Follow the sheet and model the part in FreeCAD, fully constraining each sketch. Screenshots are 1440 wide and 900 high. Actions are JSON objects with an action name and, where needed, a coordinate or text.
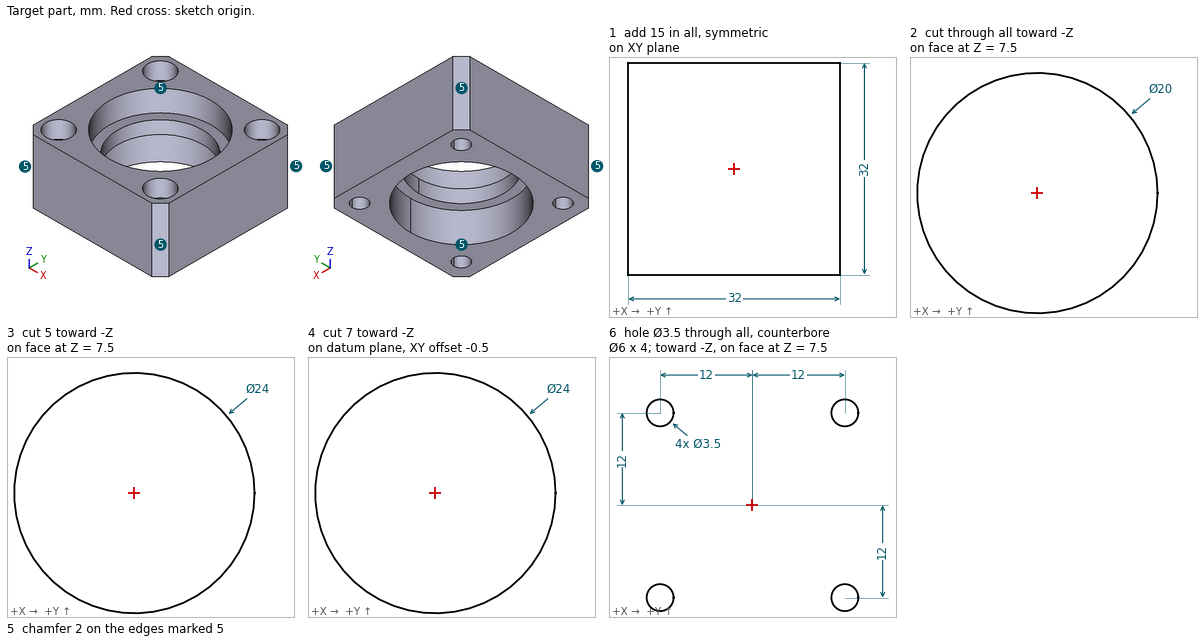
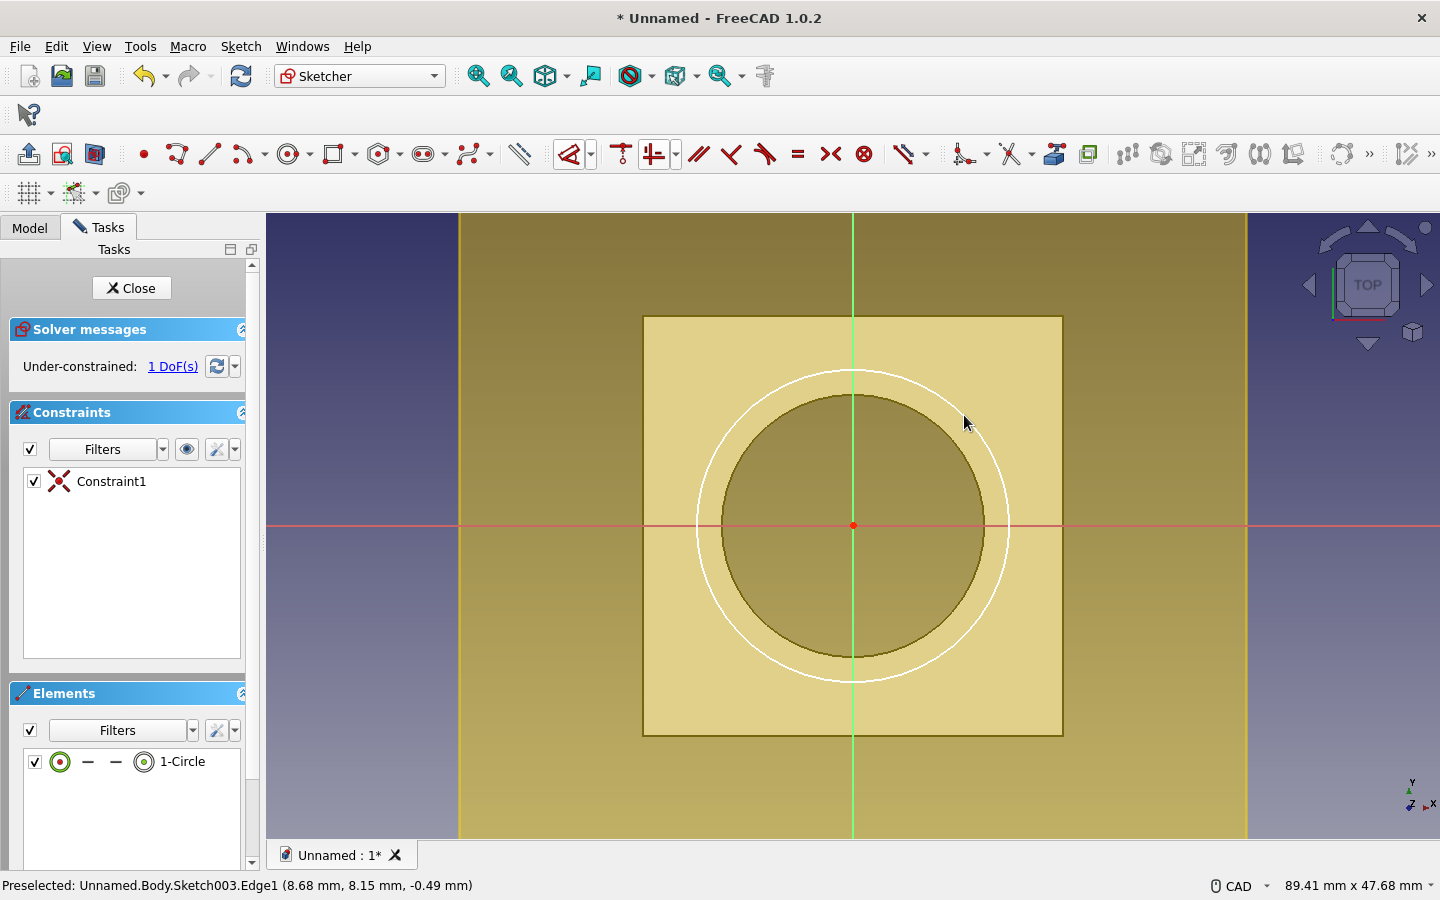
{"action": "left_click", "coordinate": [963, 415]}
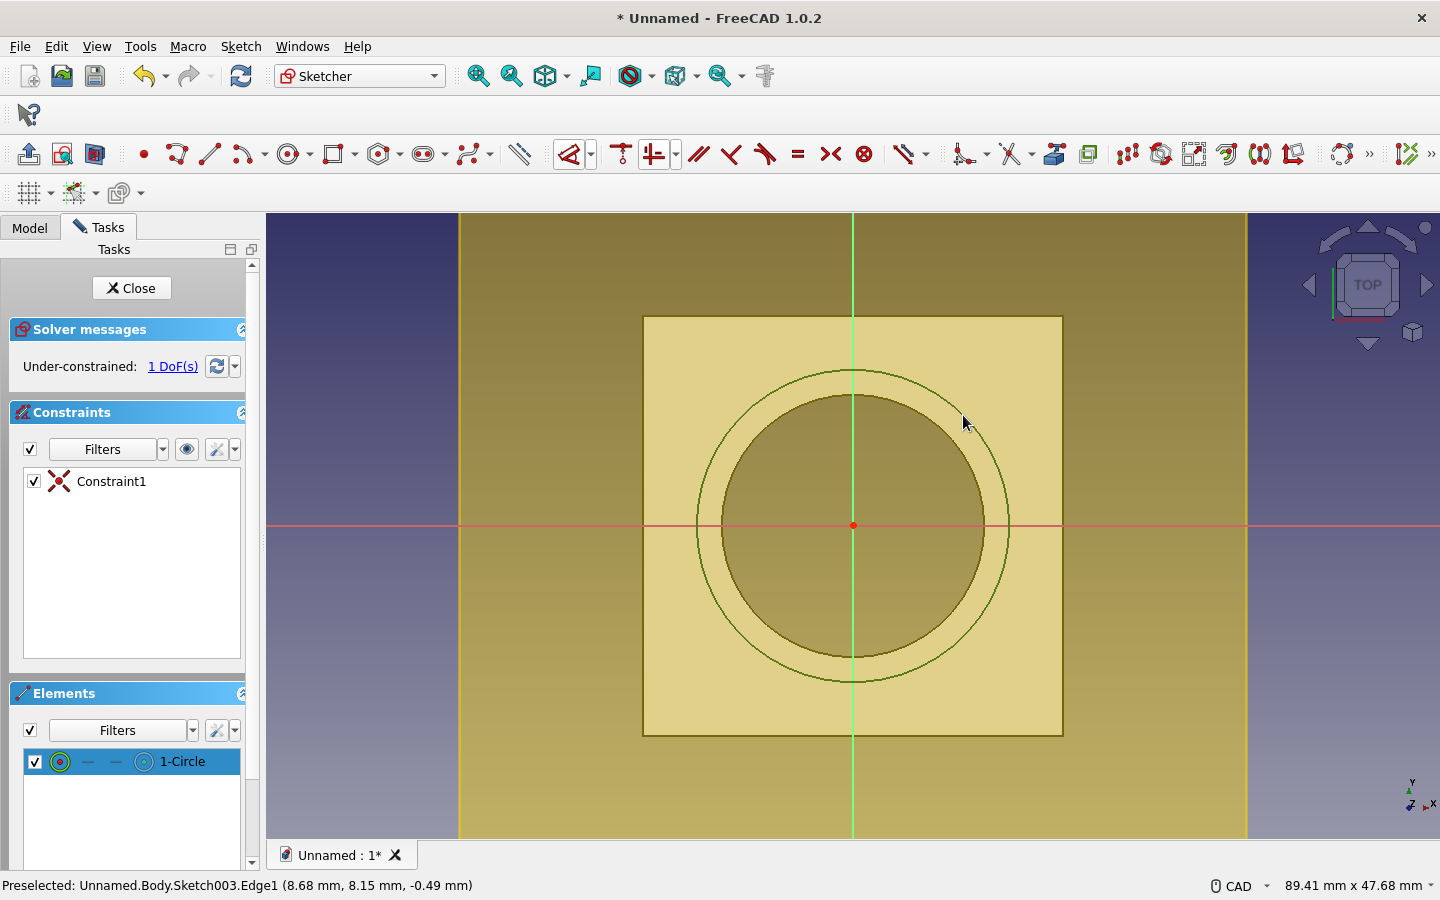
{"action": "key", "text": "k o"}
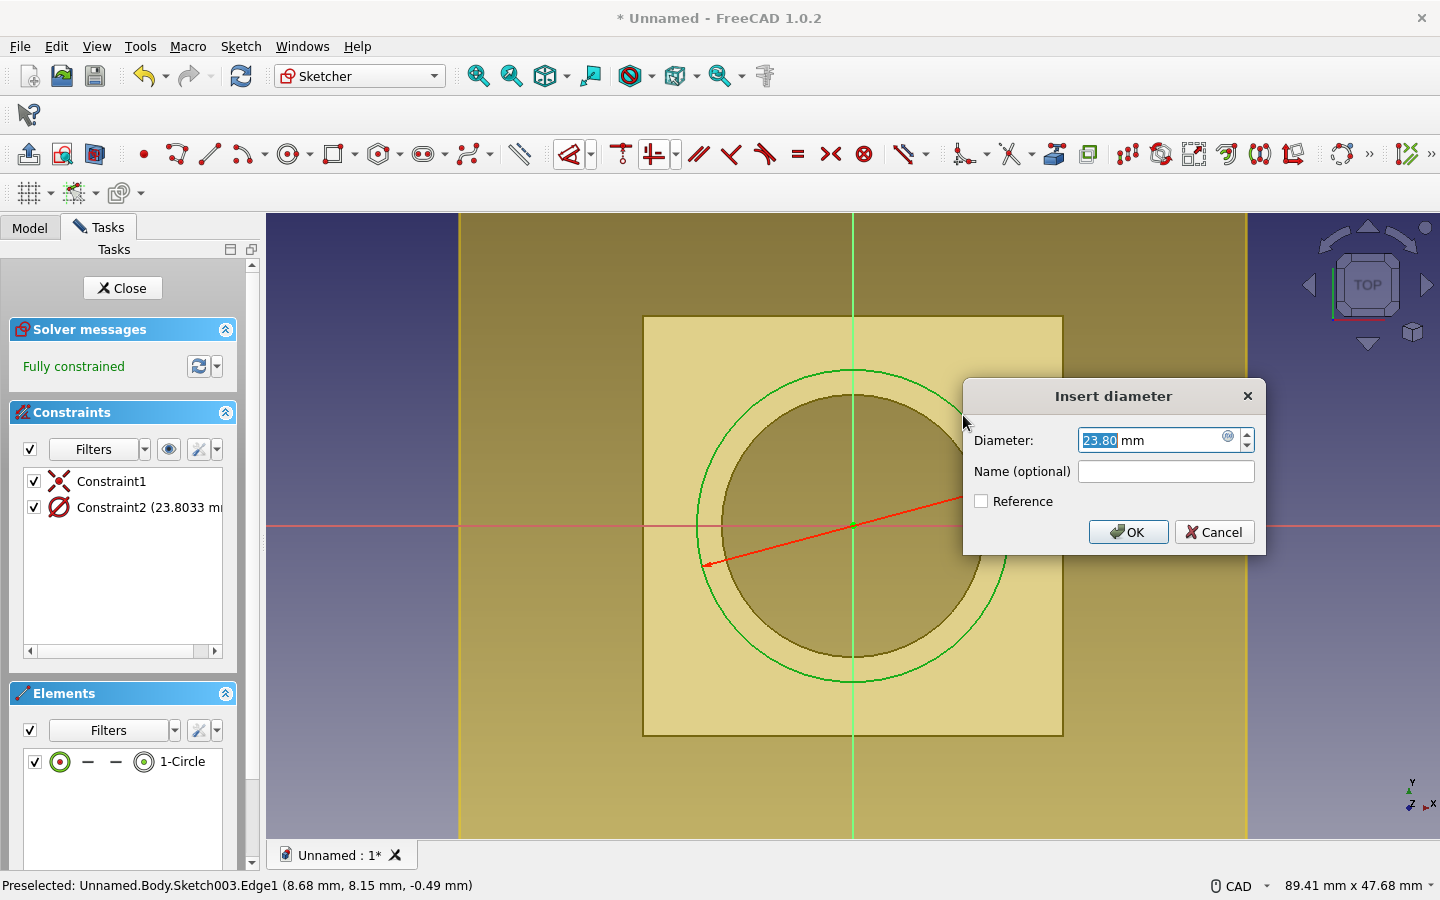
{"action": "type", "text": "24"}
{"action": "key", "text": "Return"}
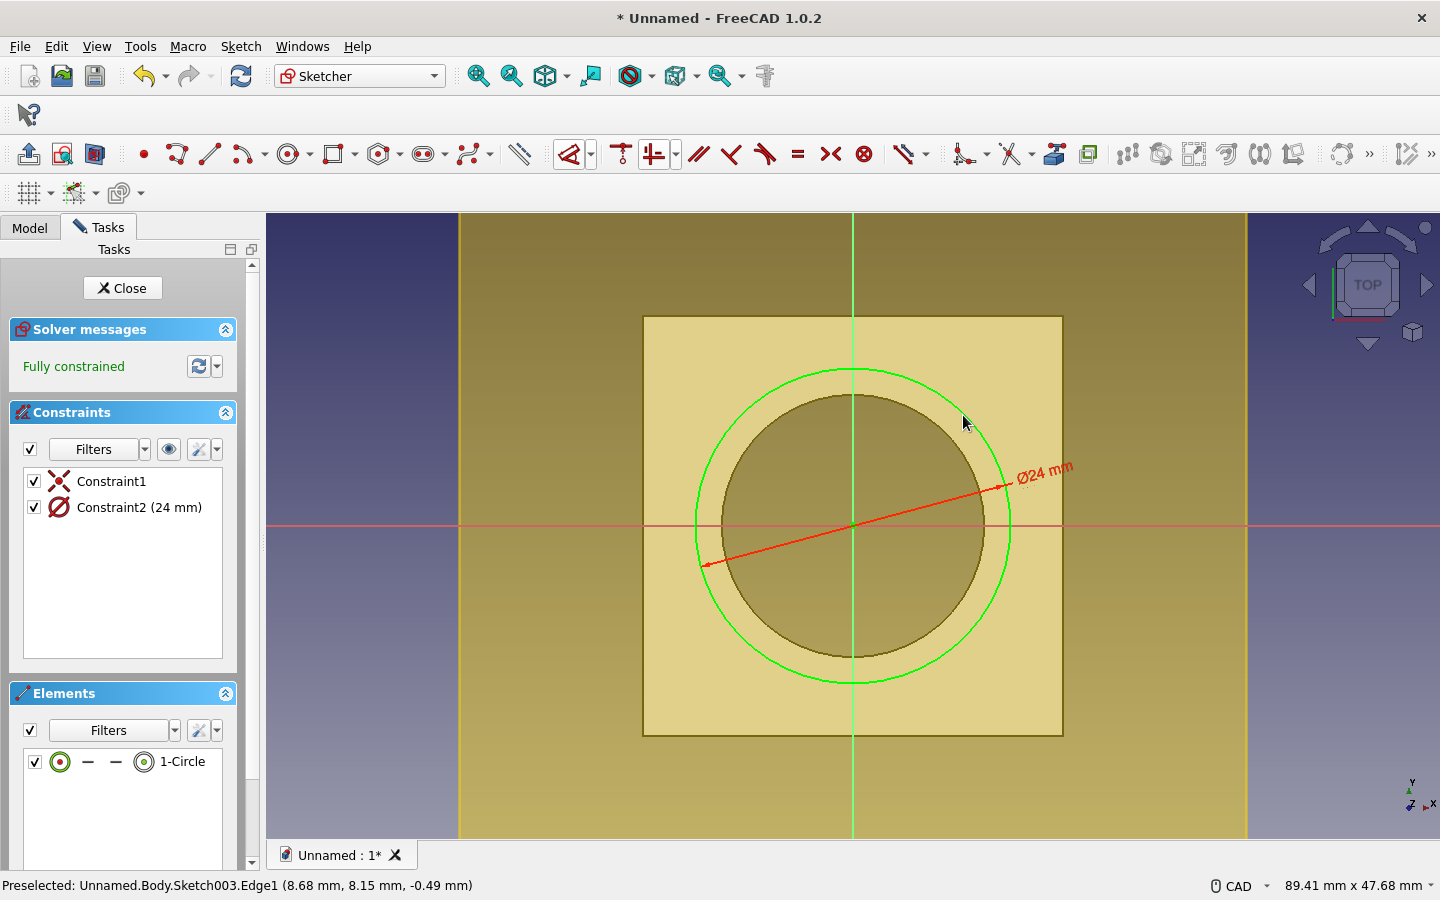
{"action": "left_click", "coordinate": [123, 288]}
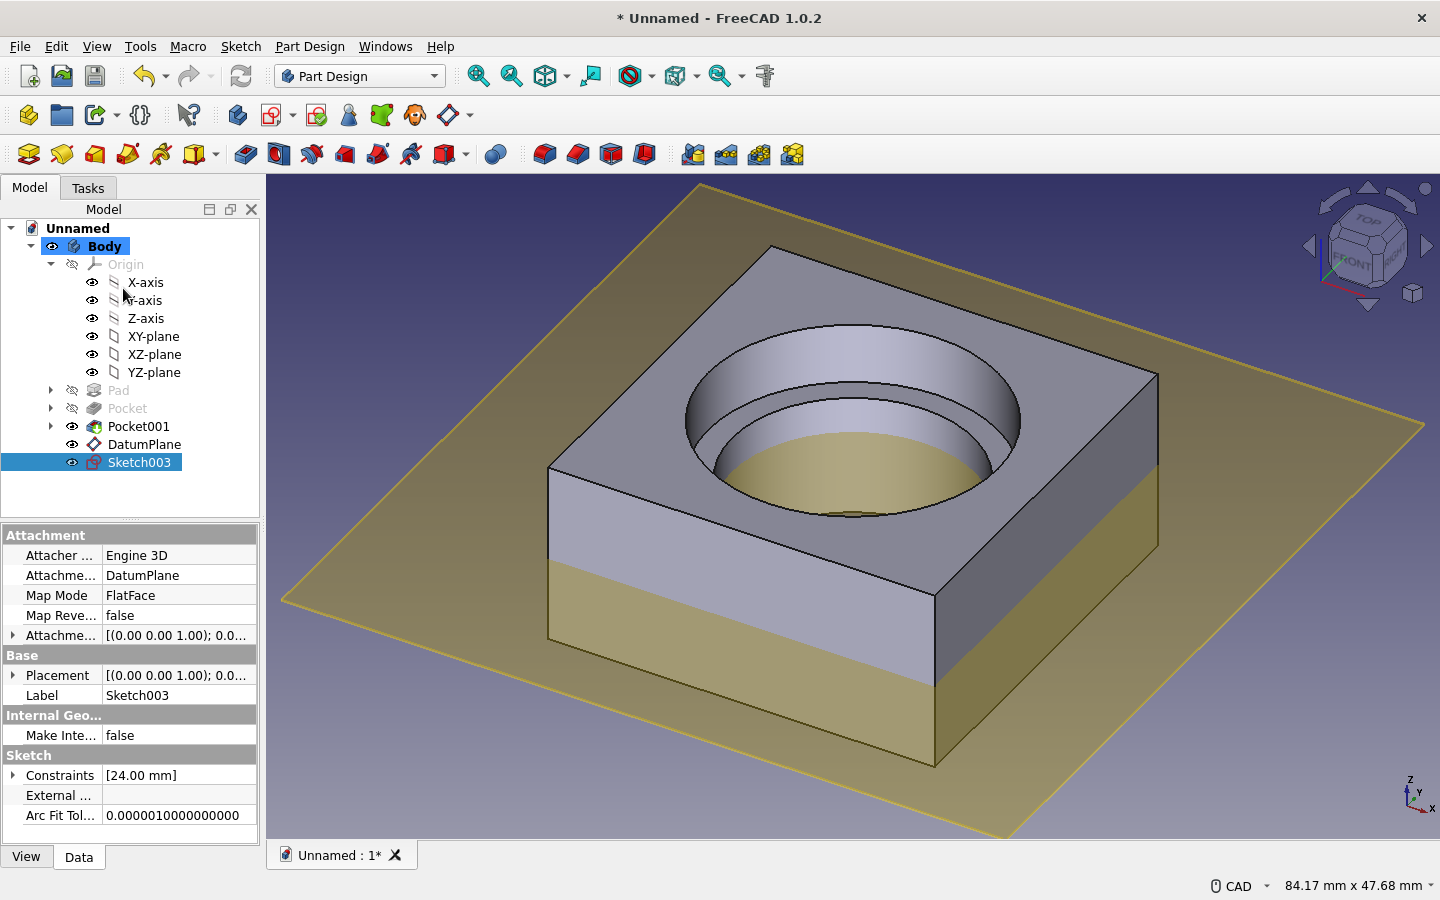
{"action": "left_click", "coordinate": [246, 154]}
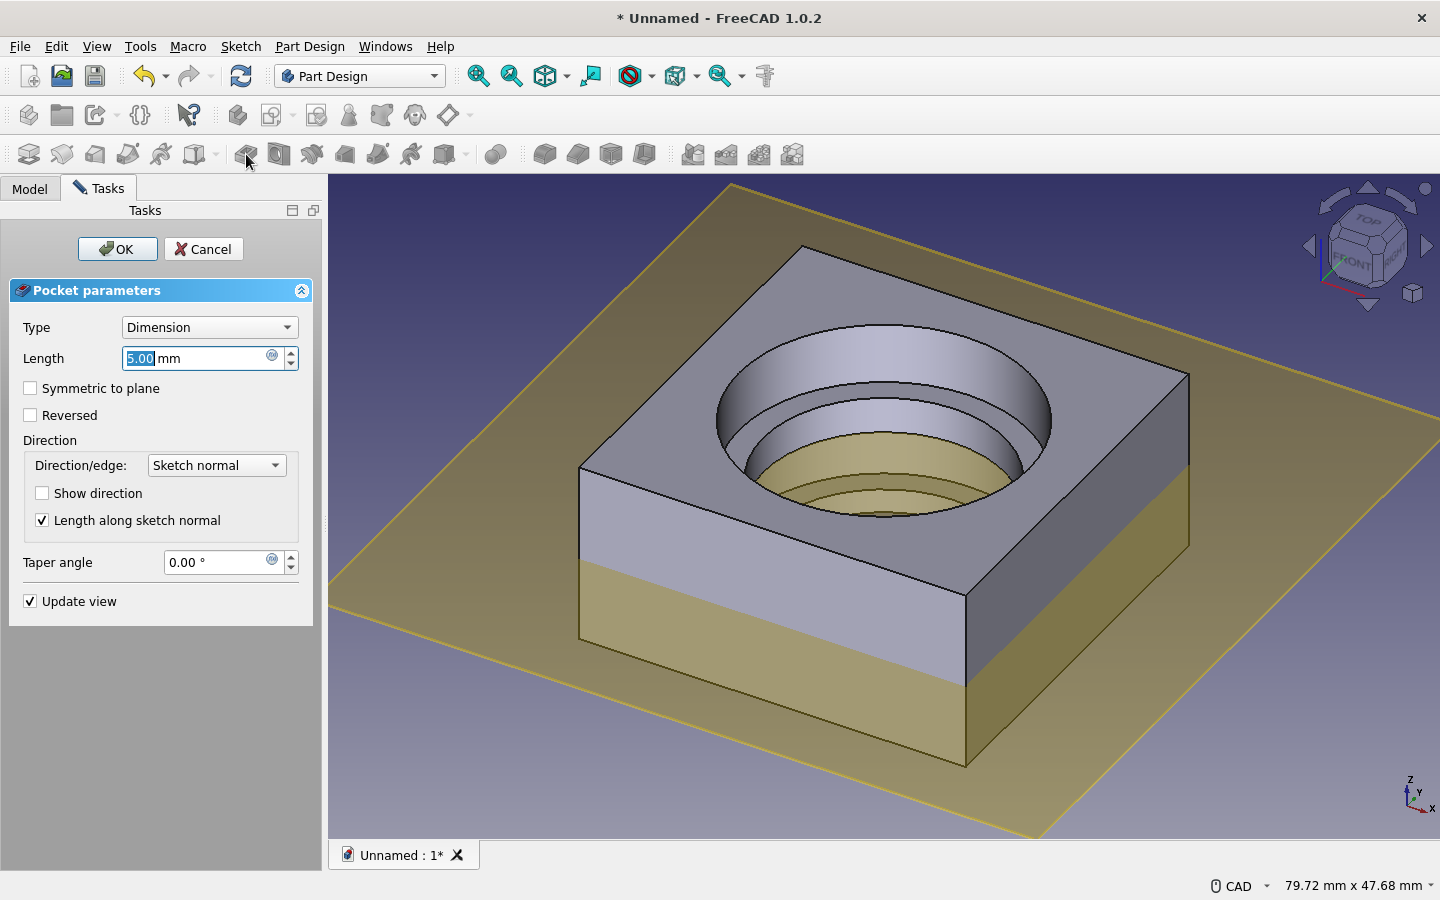
{"action": "type", "text": "7"}
{"action": "key", "text": "Tab"}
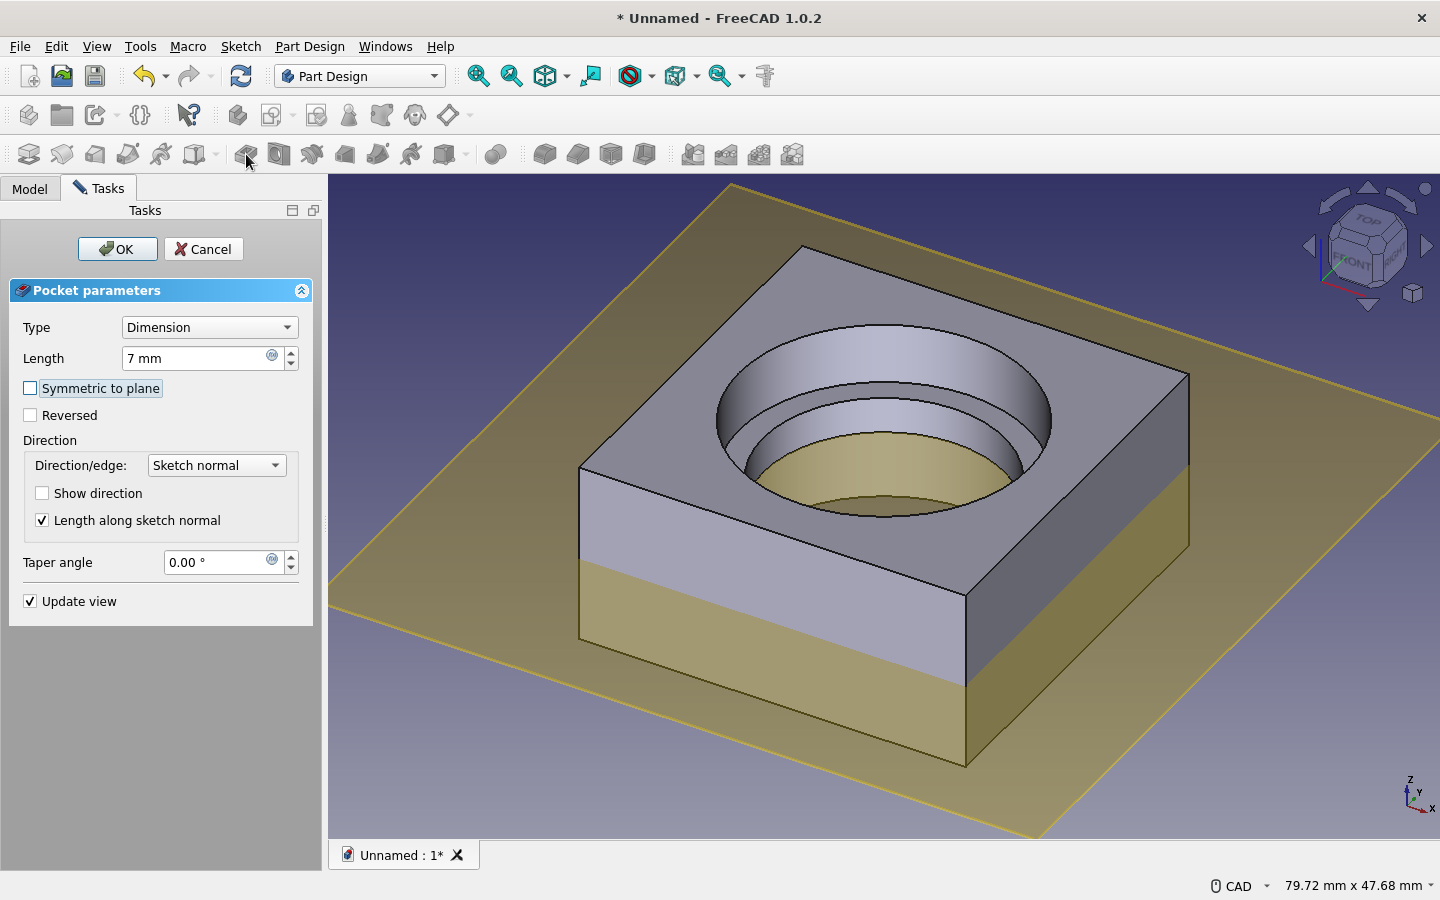
{"action": "left_click", "coordinate": [118, 249]}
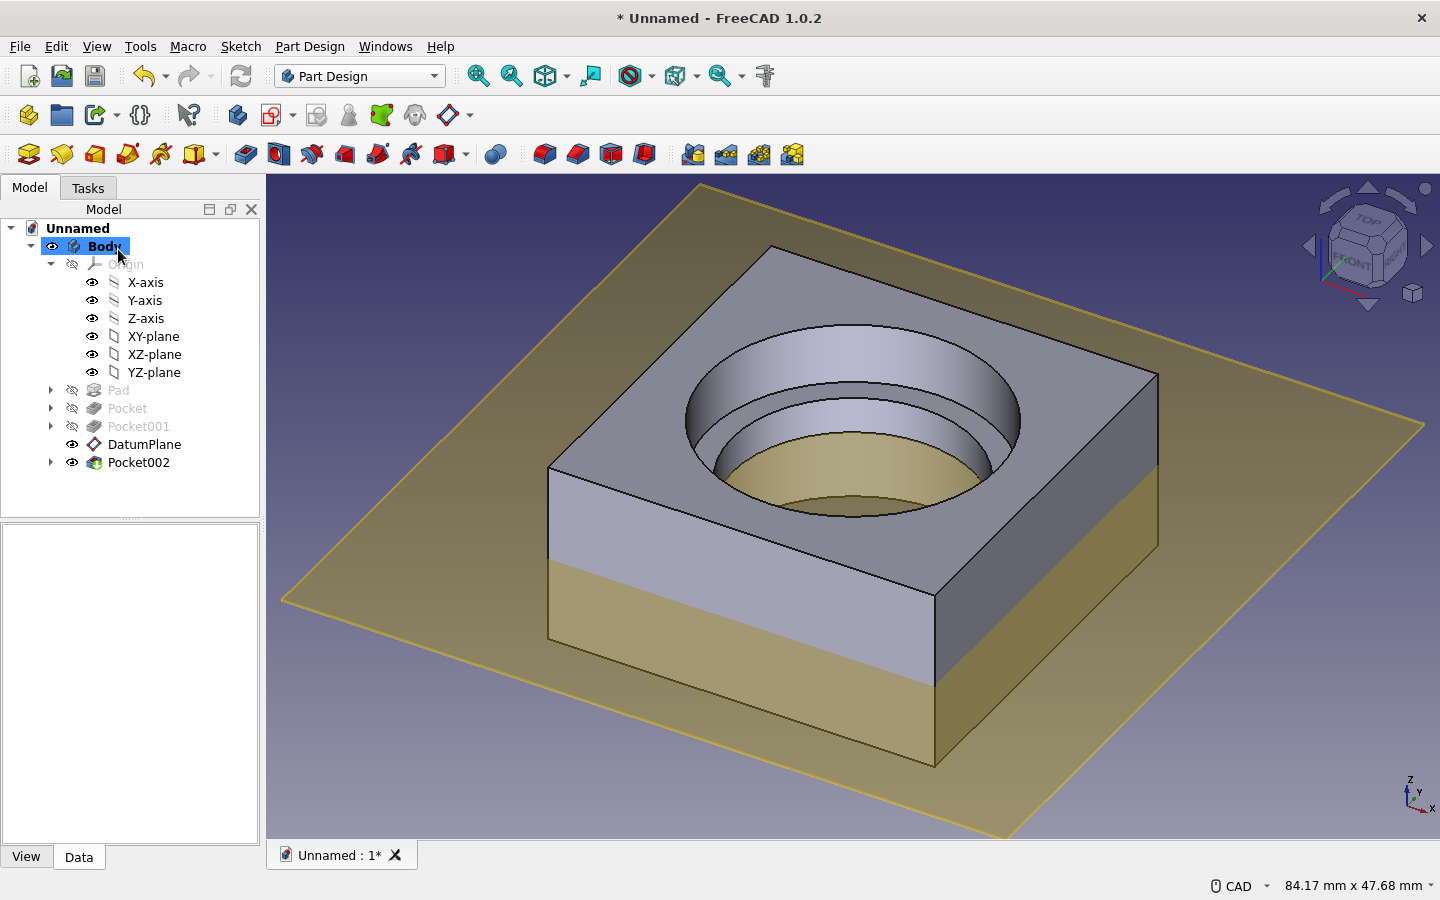
{"action": "left_click", "coordinate": [117, 444]}
{"action": "key", "text": "space"}